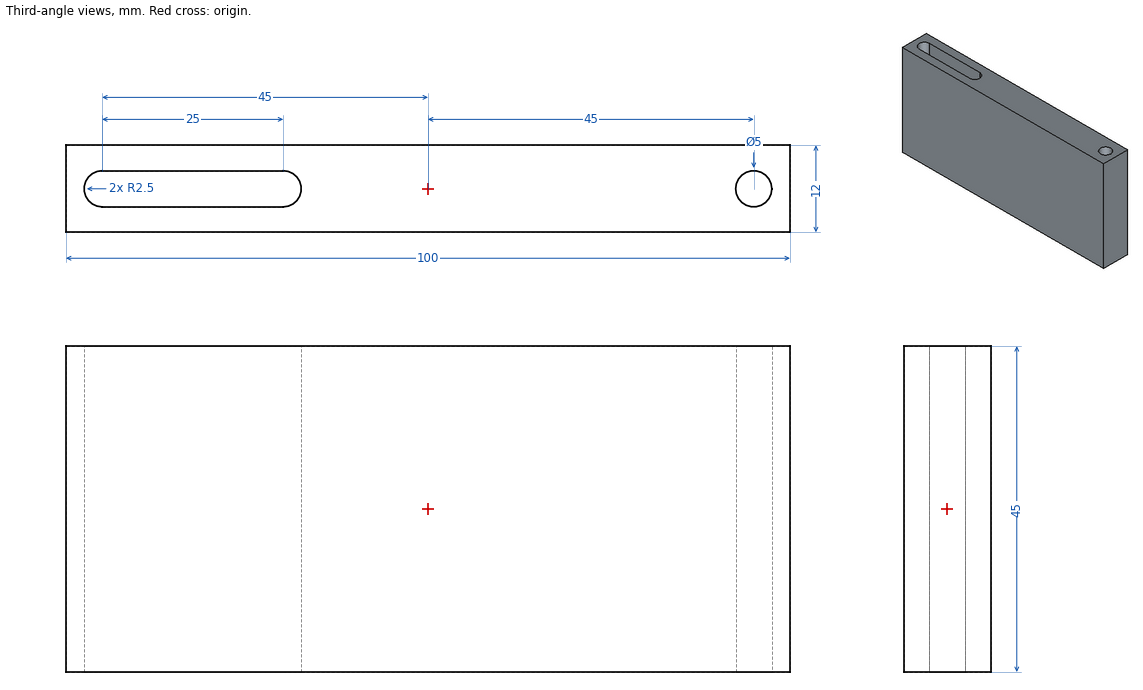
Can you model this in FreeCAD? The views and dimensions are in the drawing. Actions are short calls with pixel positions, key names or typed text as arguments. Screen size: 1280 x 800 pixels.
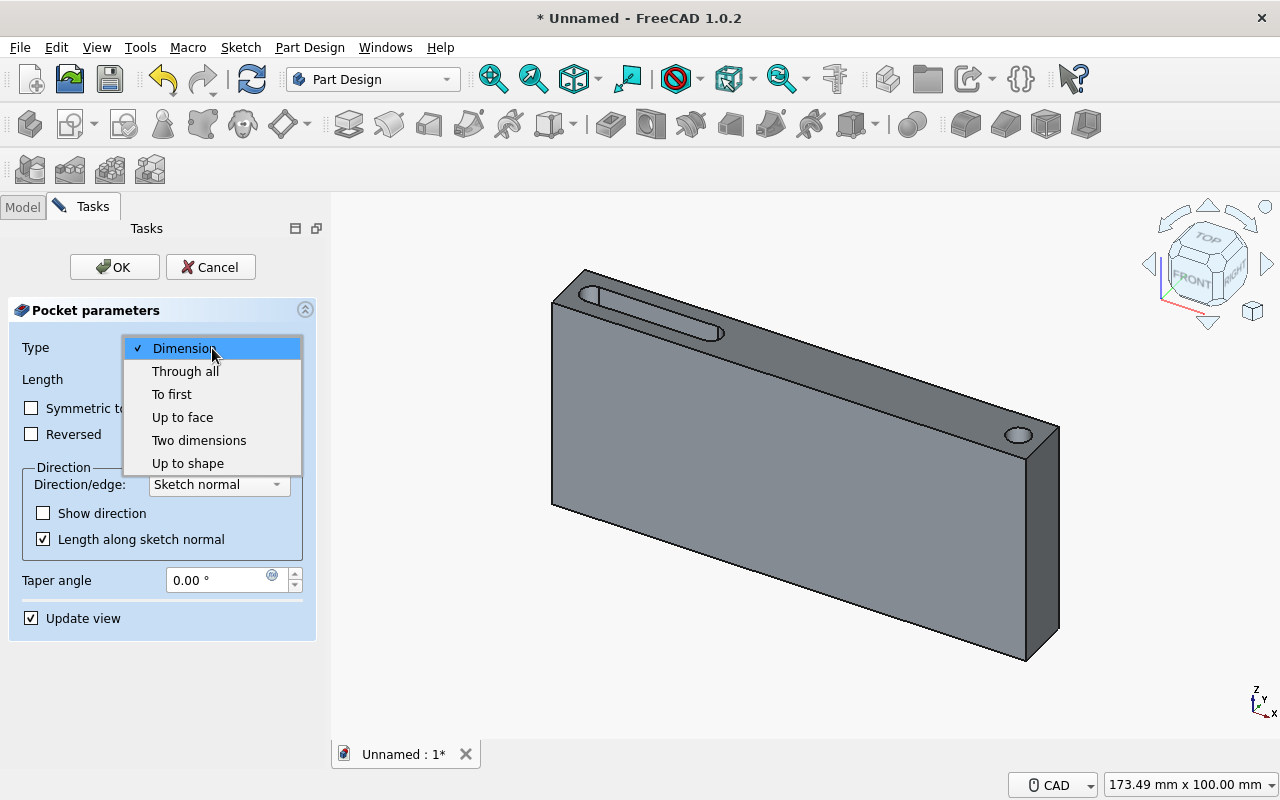
click(212, 394)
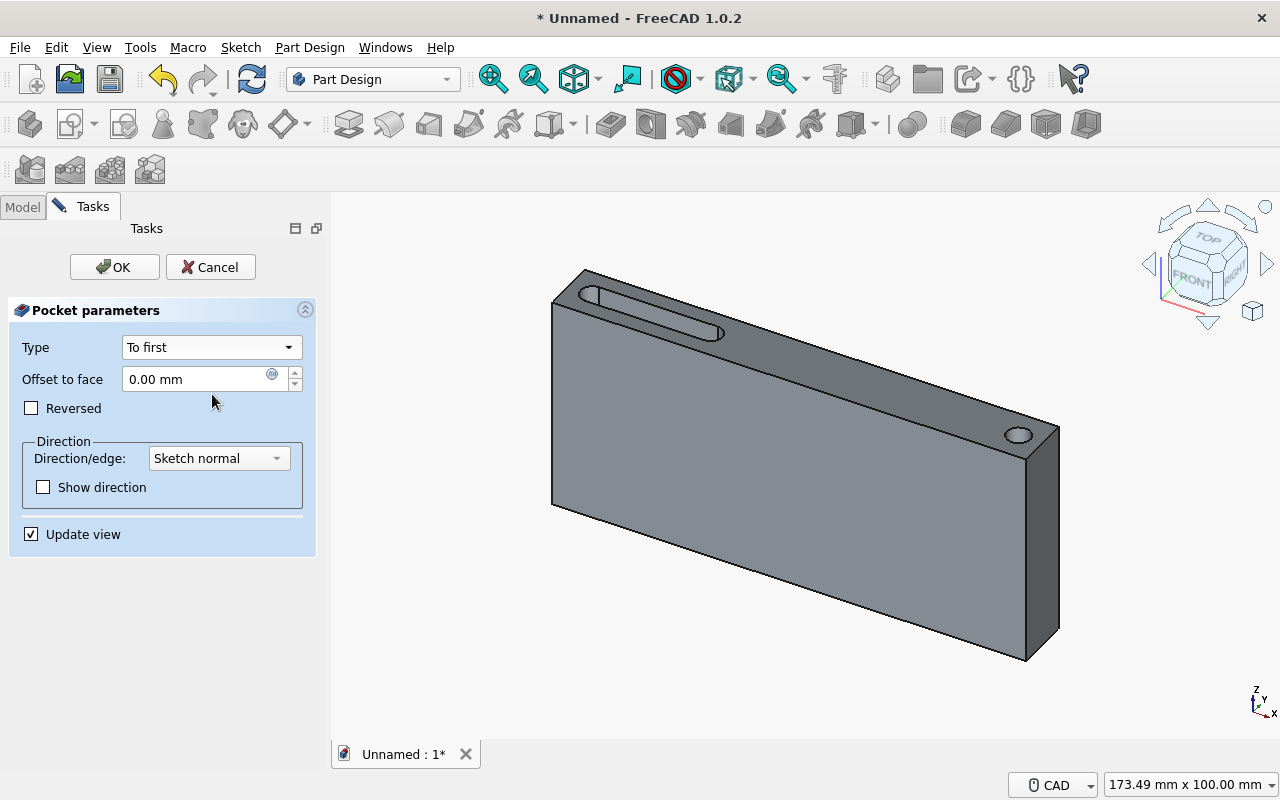
click(115, 267)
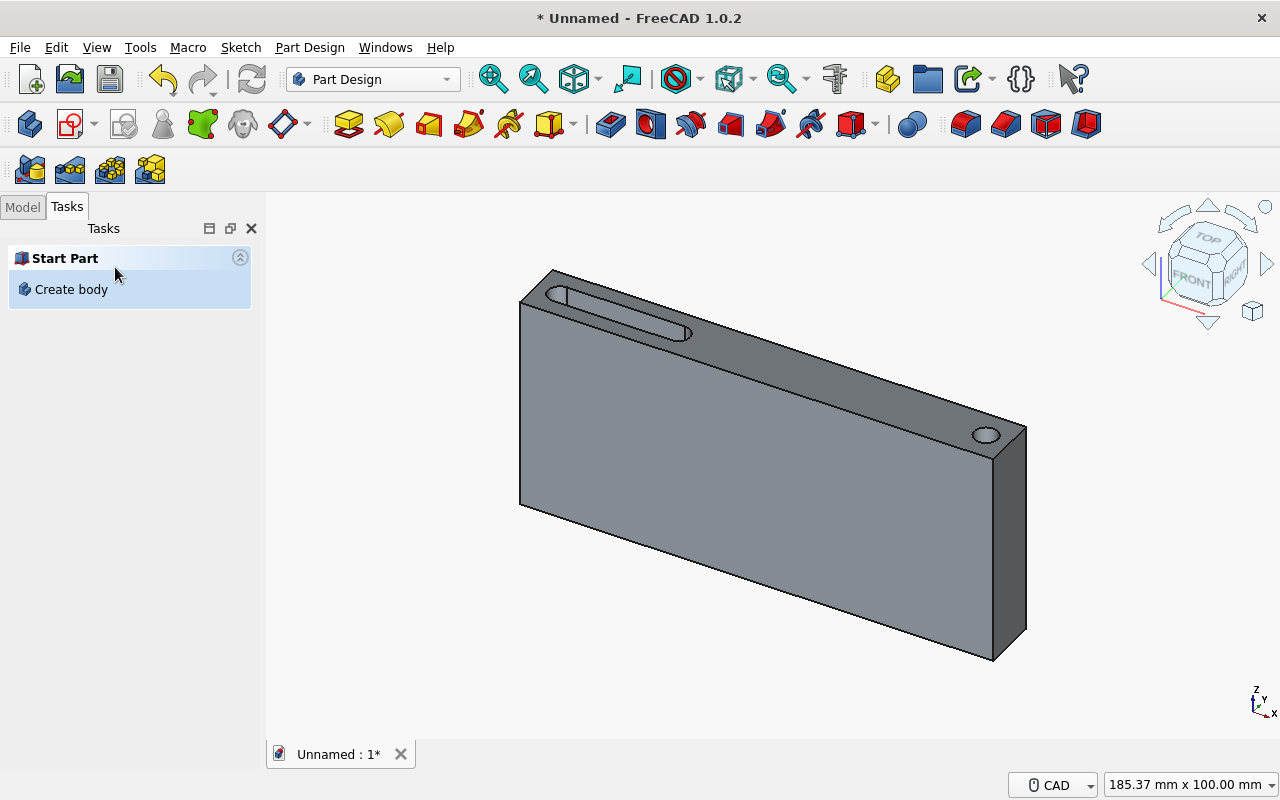
key(0)